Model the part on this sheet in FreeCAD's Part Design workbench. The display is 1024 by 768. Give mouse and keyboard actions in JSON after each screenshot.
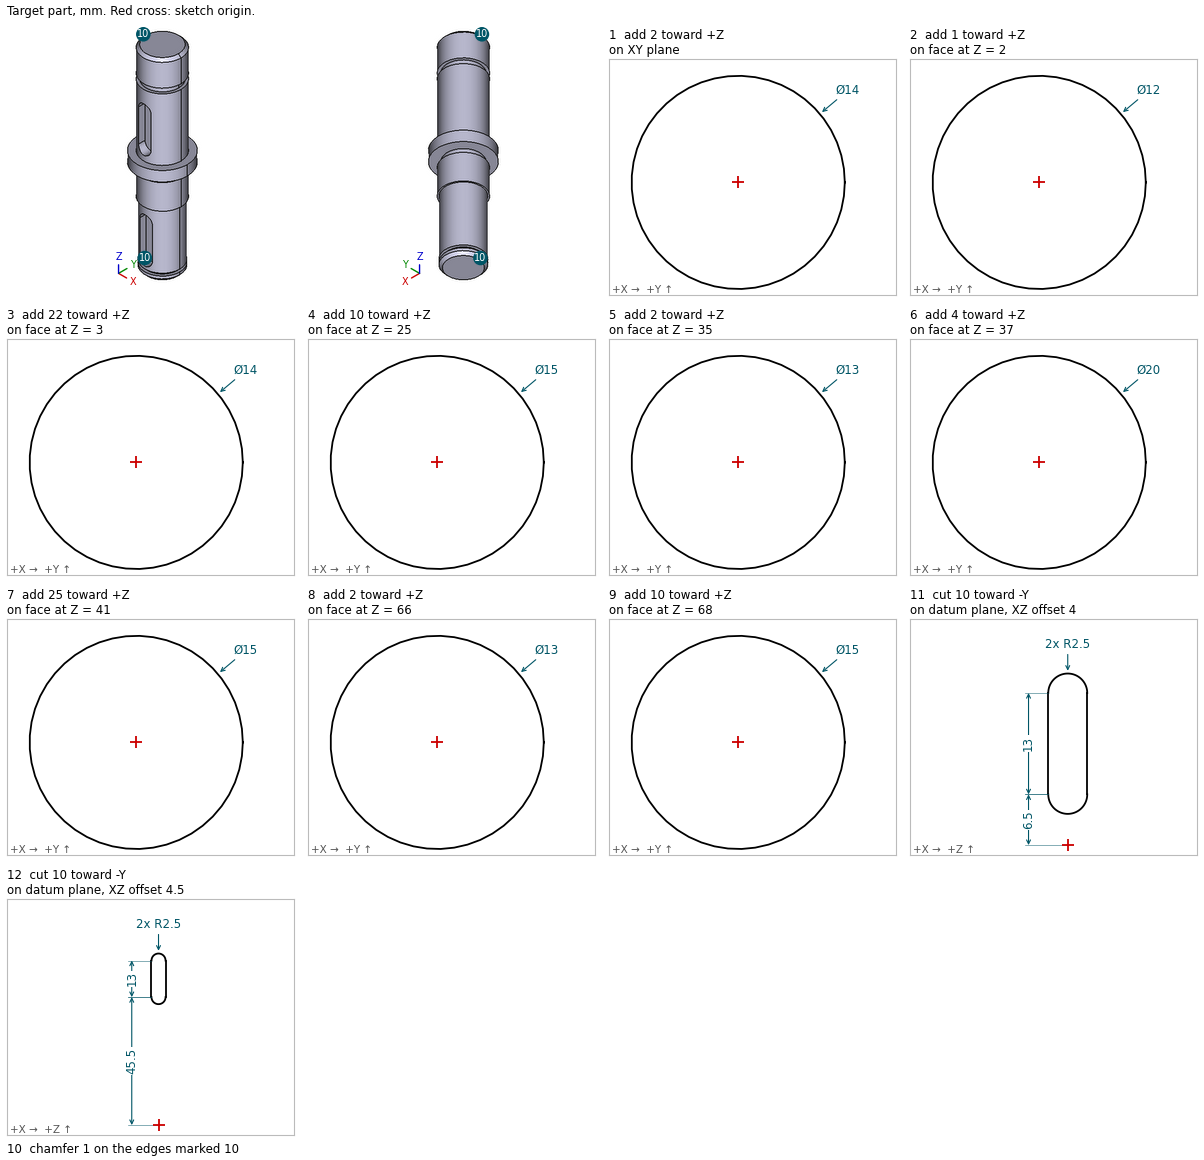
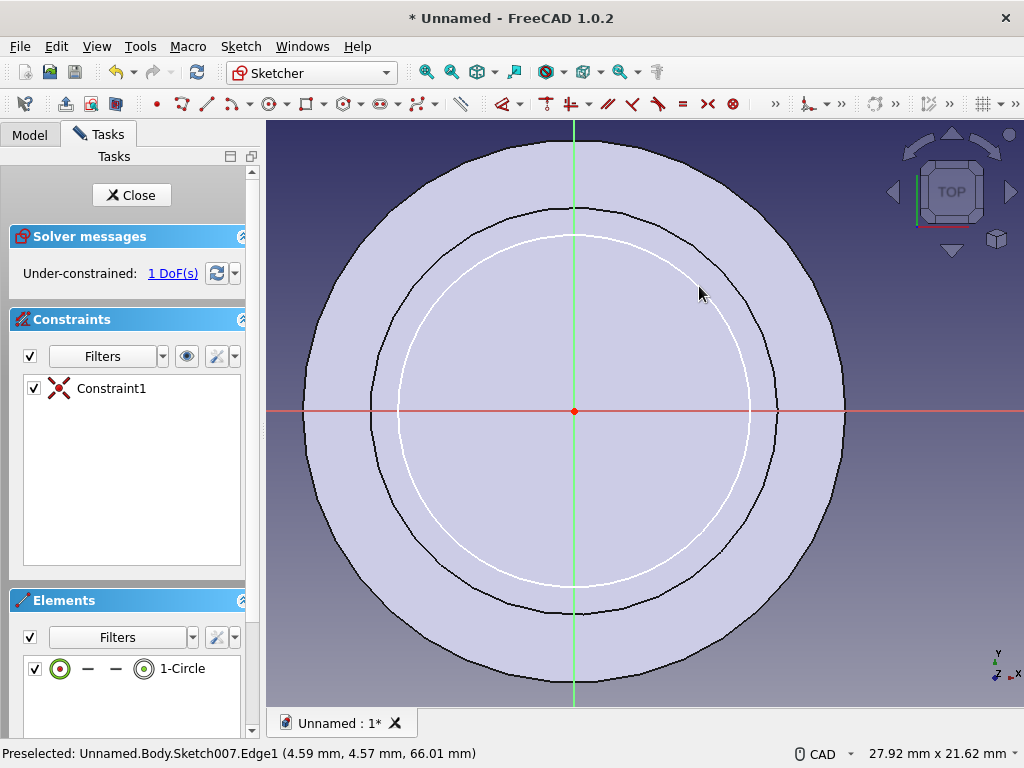
{"action": "left_click", "coordinate": [502, 104]}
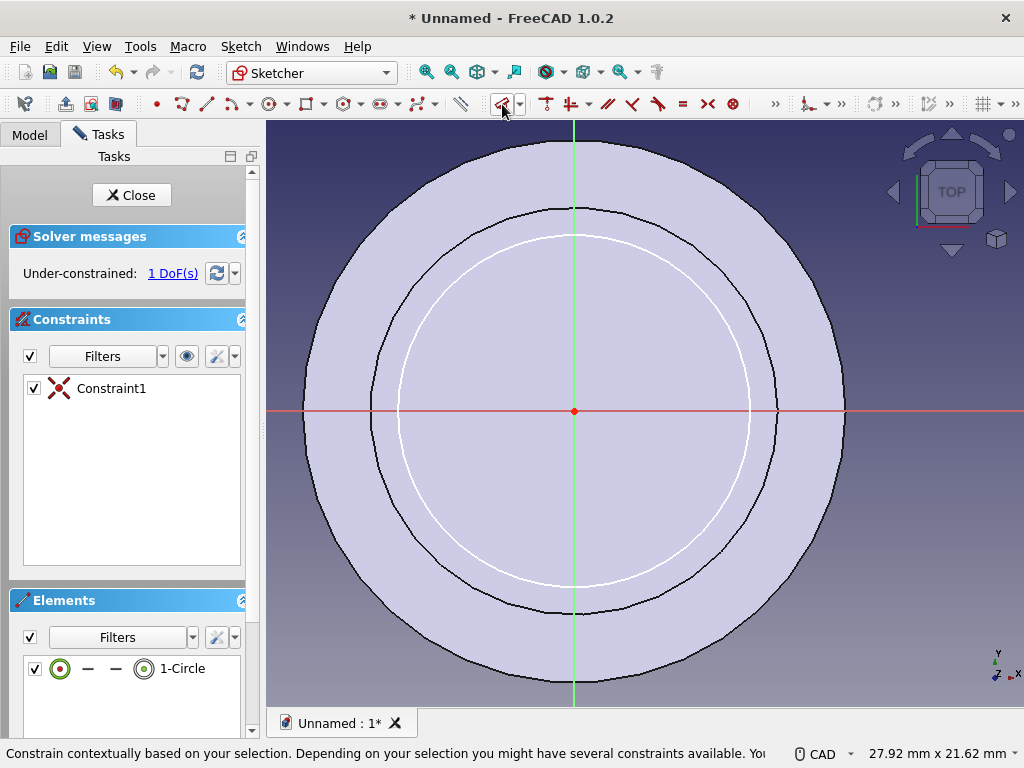
{"action": "left_click", "coordinate": [698, 286]}
{"action": "left_click", "coordinate": [721, 263]}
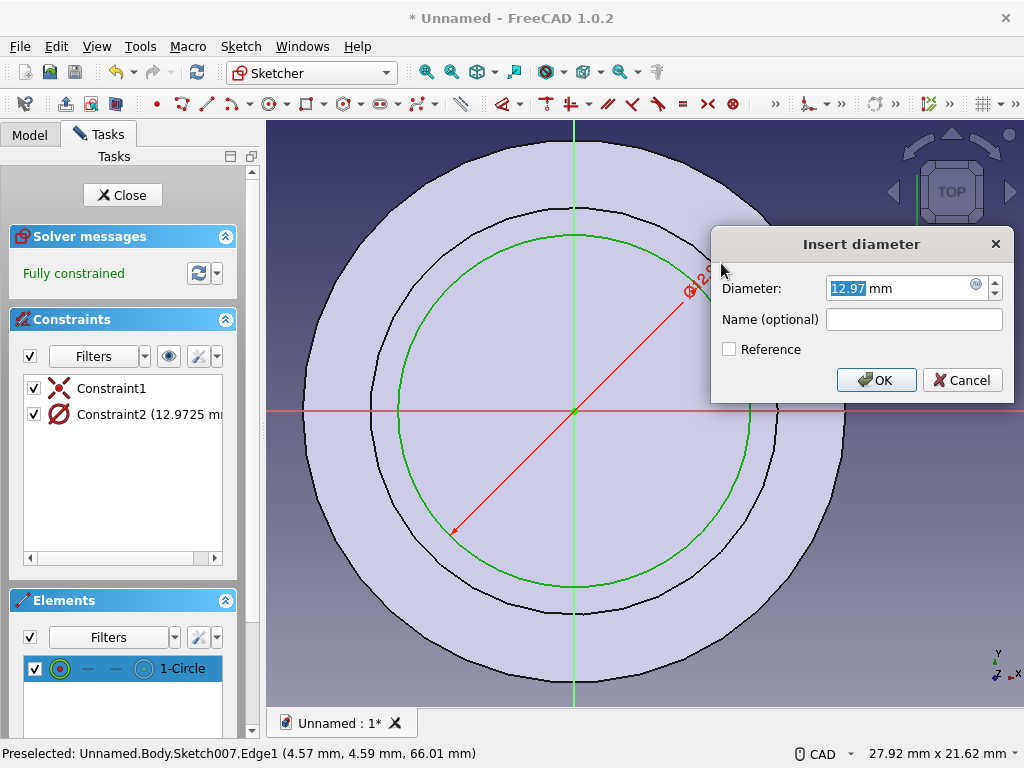
{"action": "type", "text": "13"}
{"action": "key", "text": "Return"}
{"action": "key", "text": "Escape"}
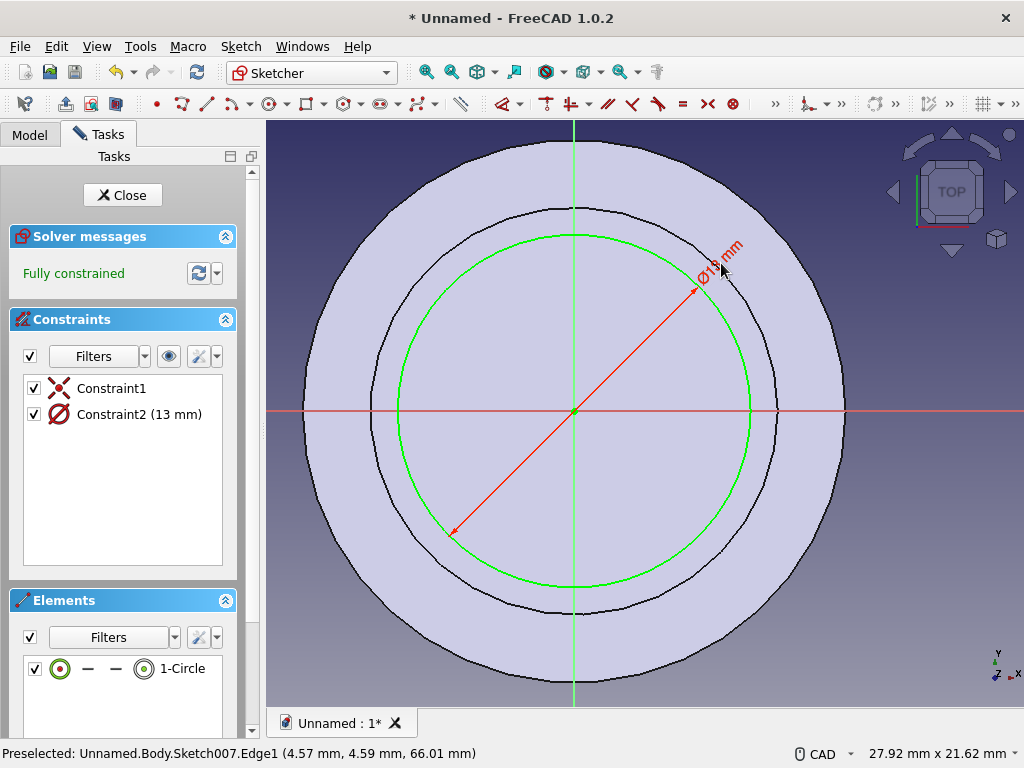
{"action": "left_click", "coordinate": [123, 195]}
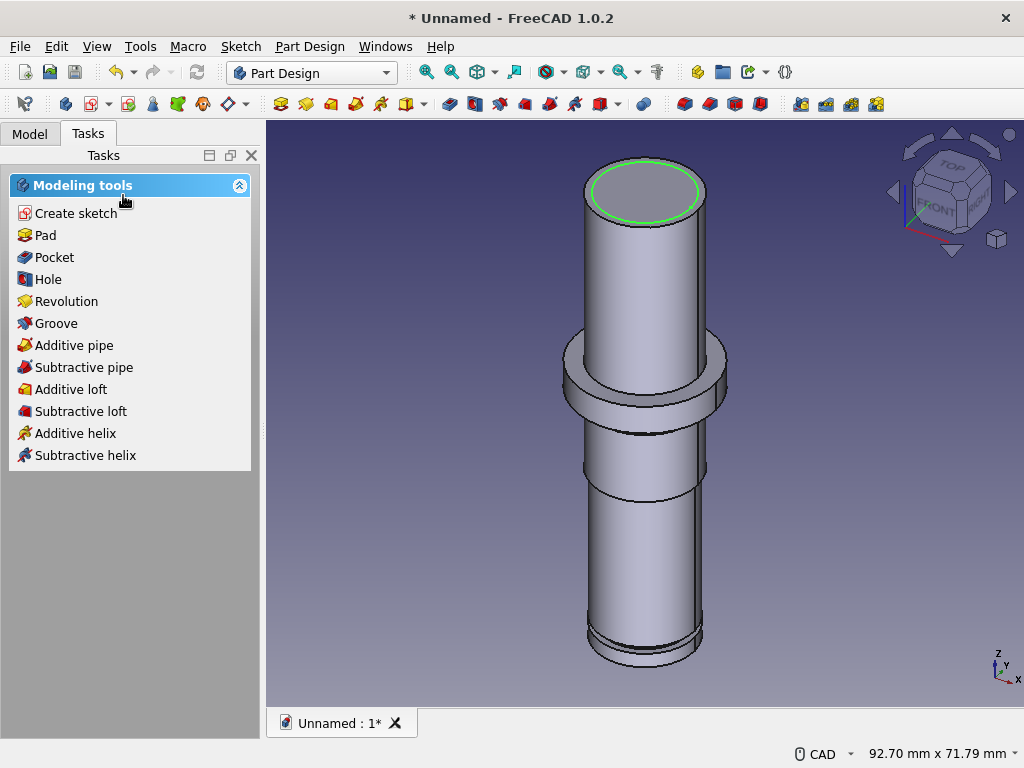
{"action": "left_click", "coordinate": [281, 104]}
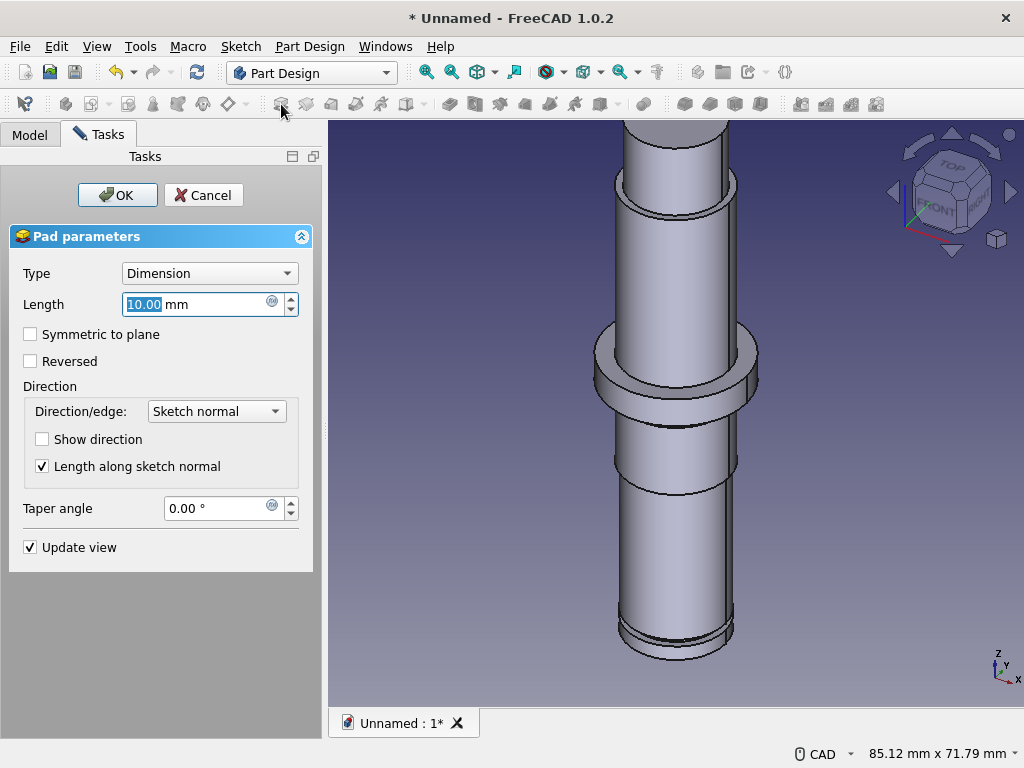
{"action": "type", "text": "2"}
{"action": "key", "text": "Tab"}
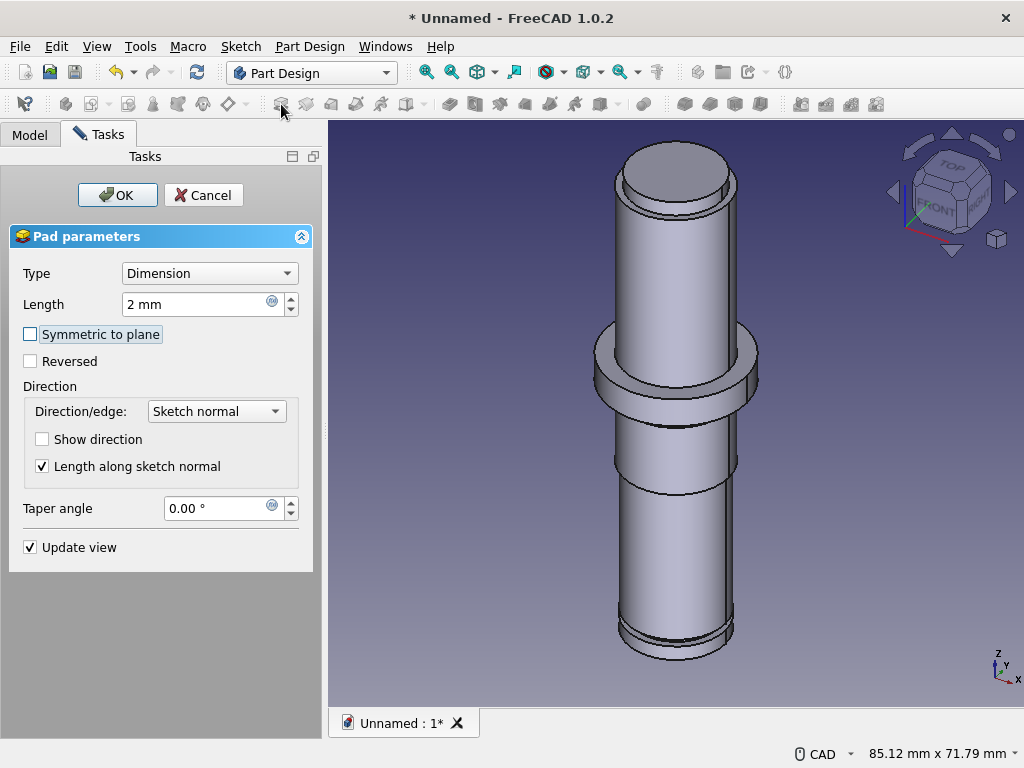
{"action": "left_click", "coordinate": [118, 195]}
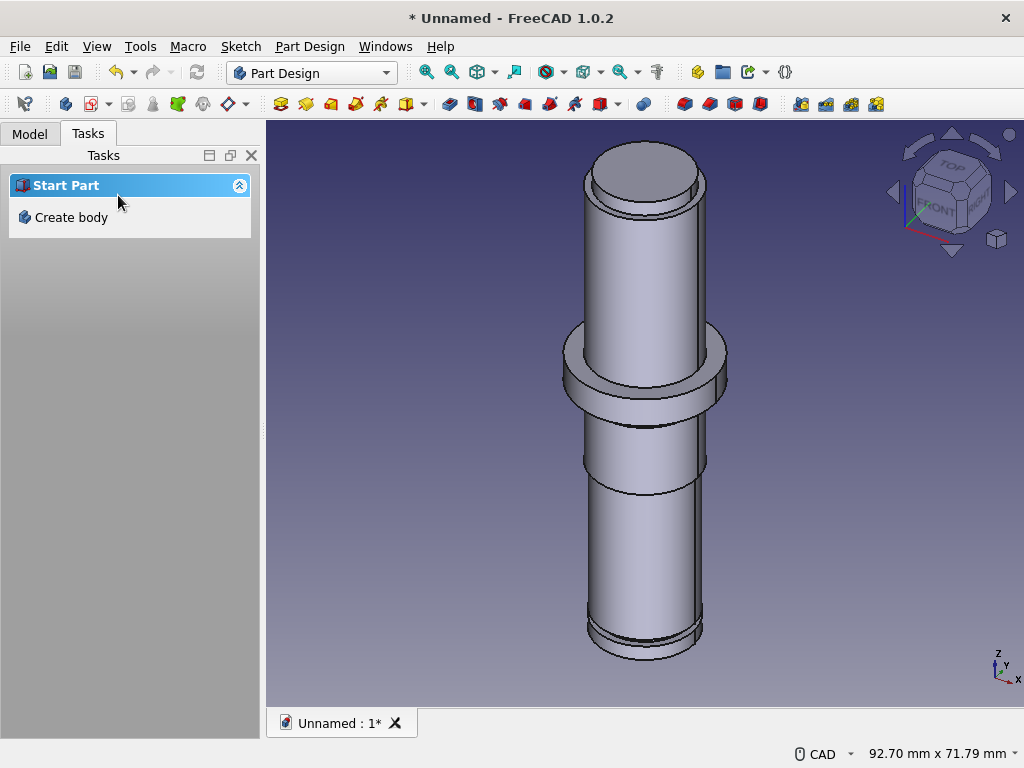
{"action": "left_click", "coordinate": [427, 72]}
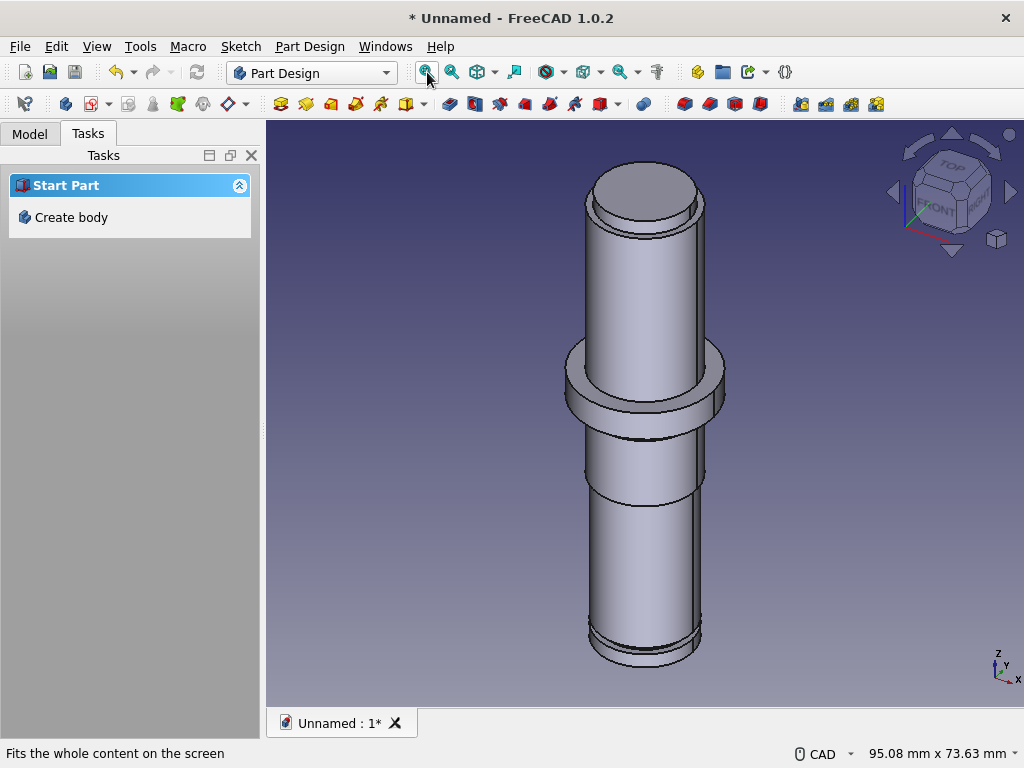
{"action": "left_click", "coordinate": [645, 190]}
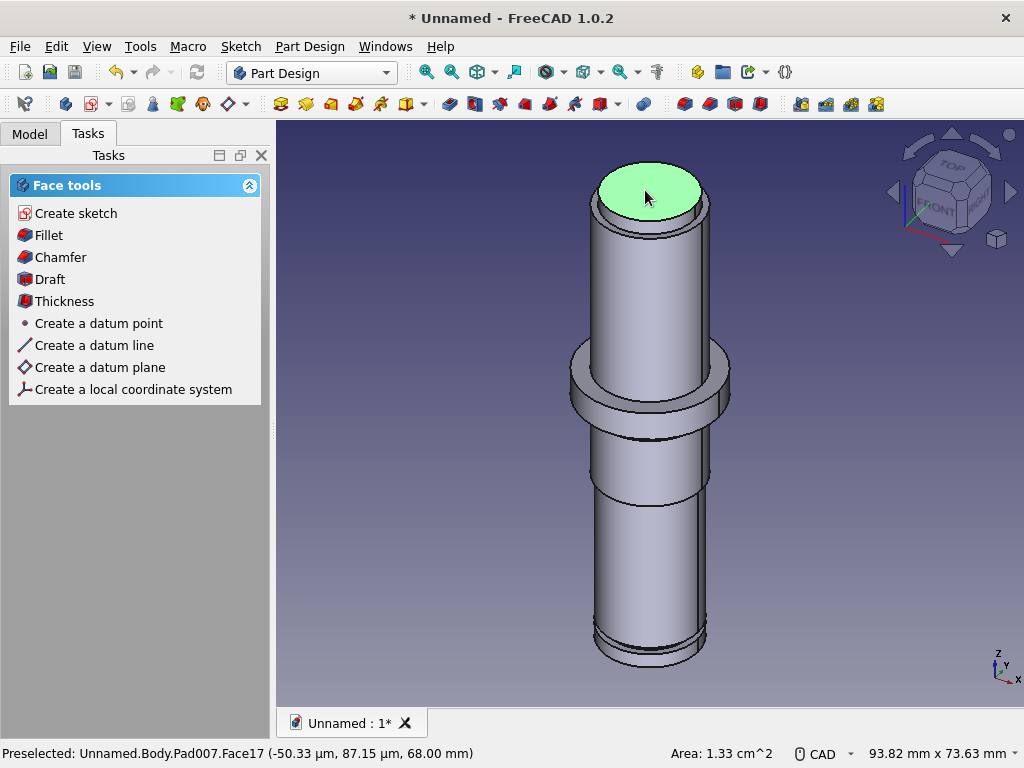
{"action": "left_click", "coordinate": [90, 104]}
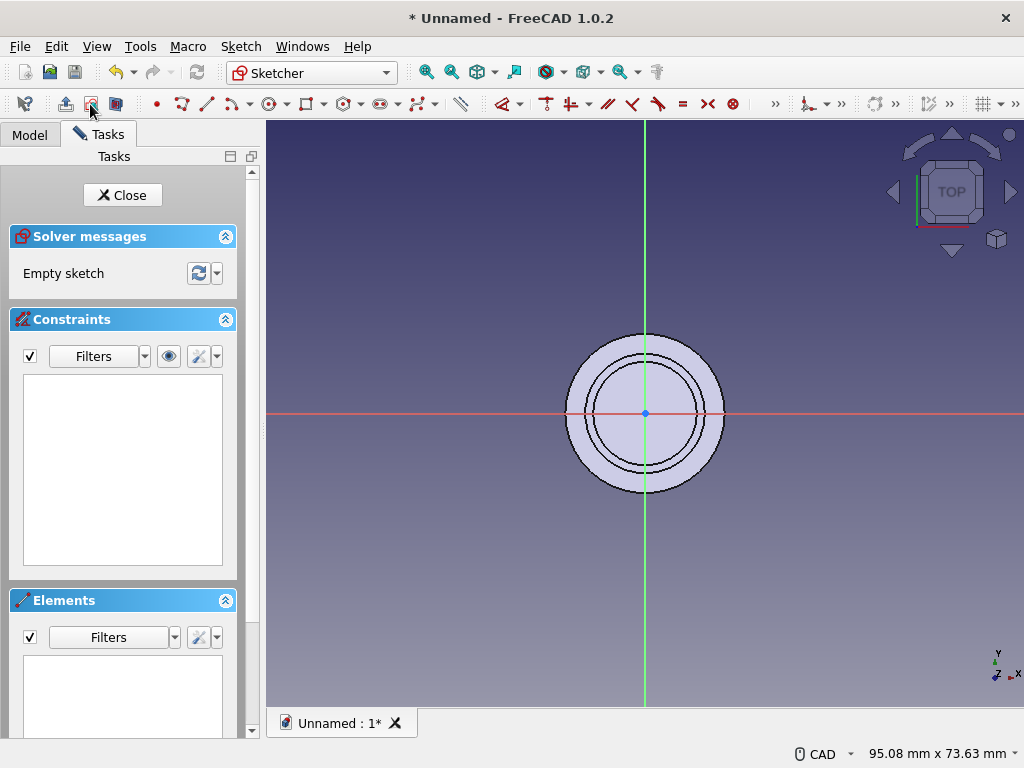
{"action": "scroll", "coordinate": [675, 414], "scroll_direction": "up", "scroll_amount": 6}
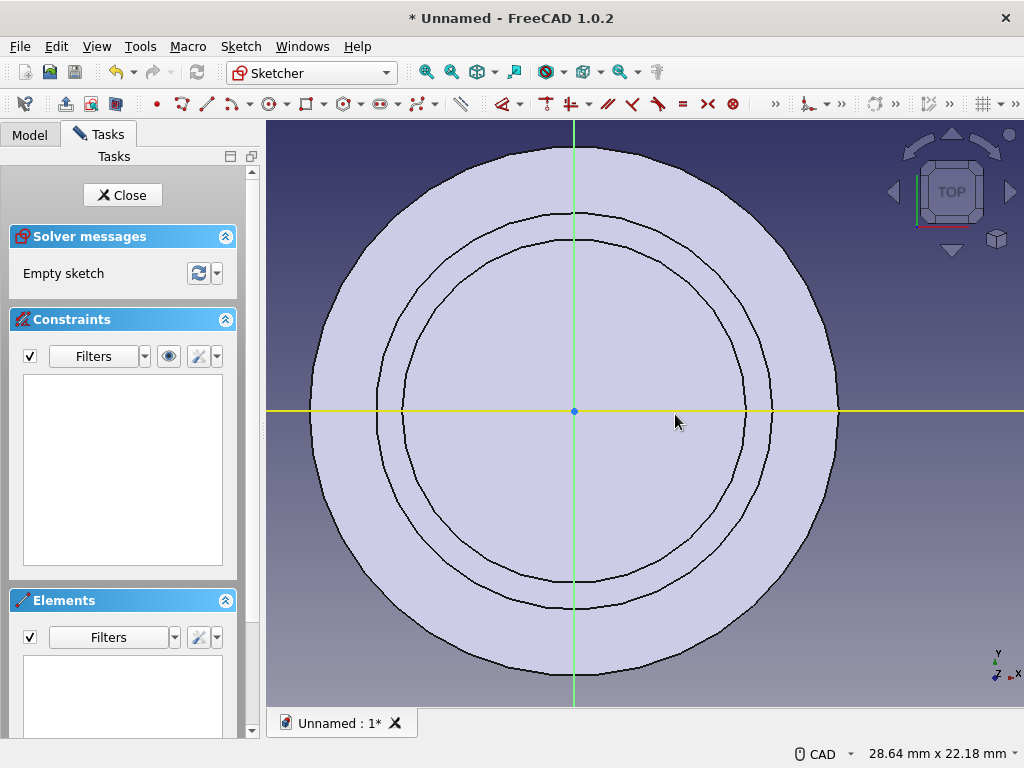
{"action": "left_click", "coordinate": [268, 104]}